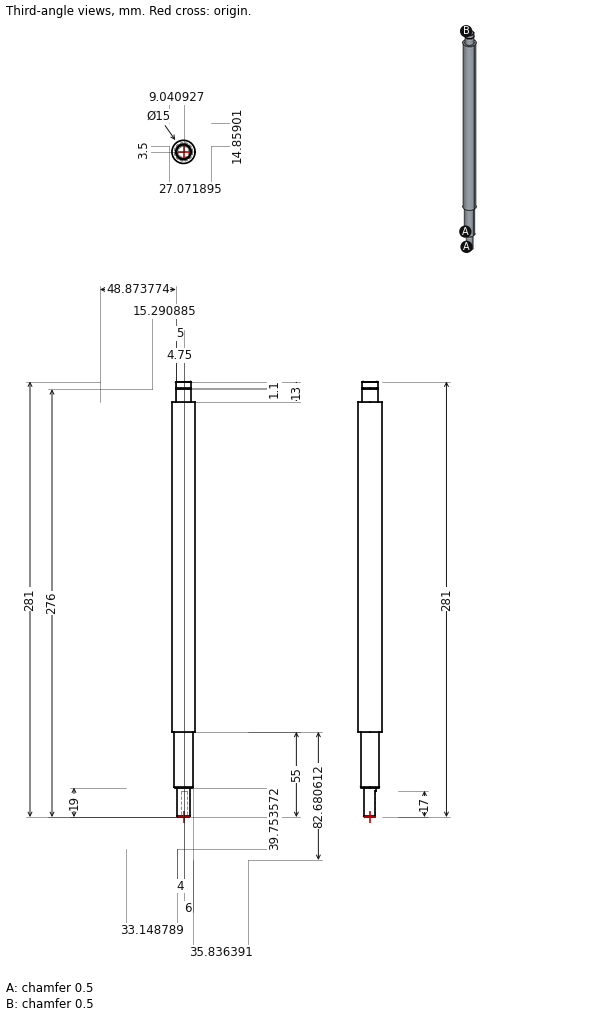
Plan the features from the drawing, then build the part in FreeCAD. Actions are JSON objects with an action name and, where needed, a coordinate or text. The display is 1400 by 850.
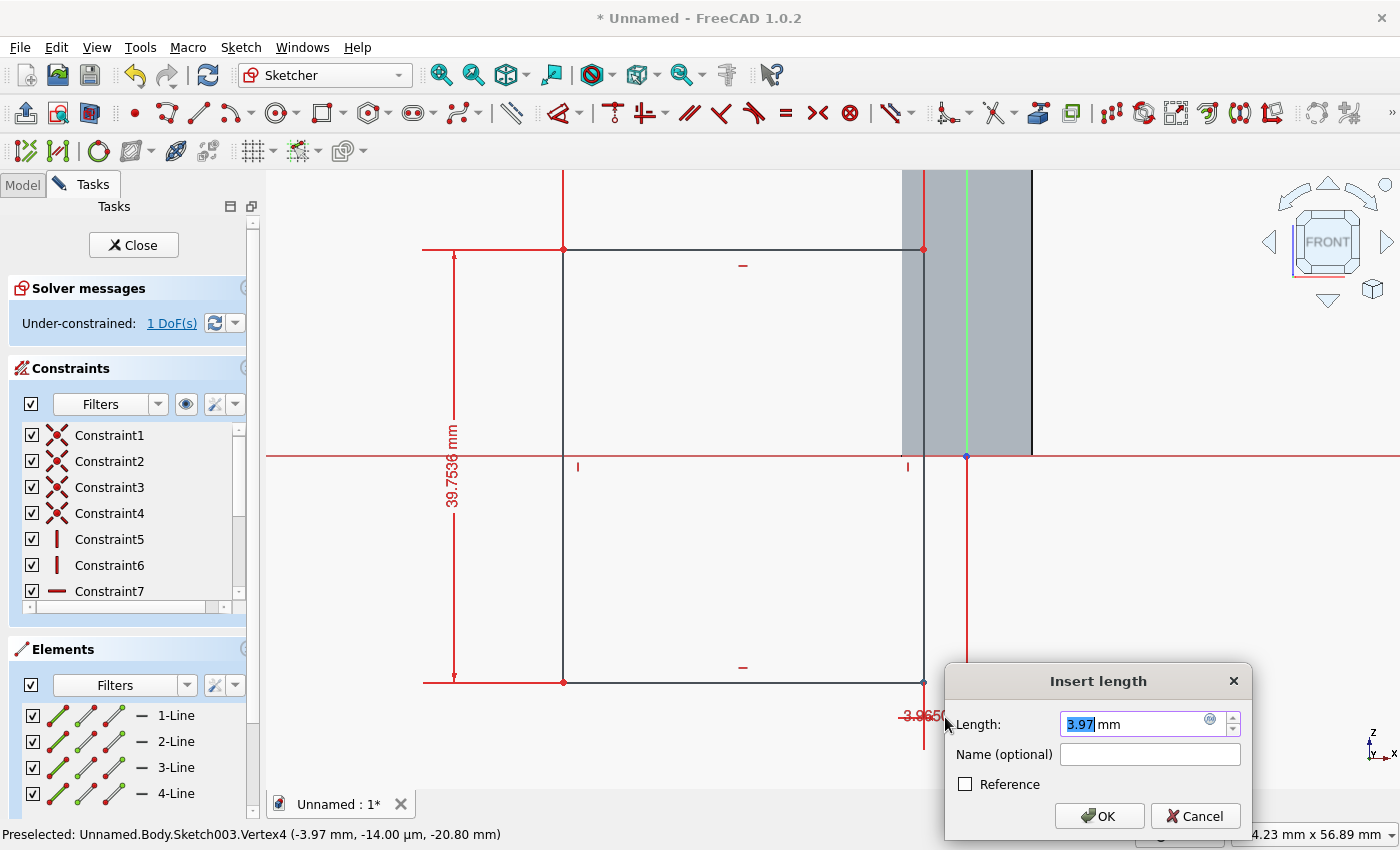
{"action": "type", "text": "4"}
{"action": "key", "text": "Return"}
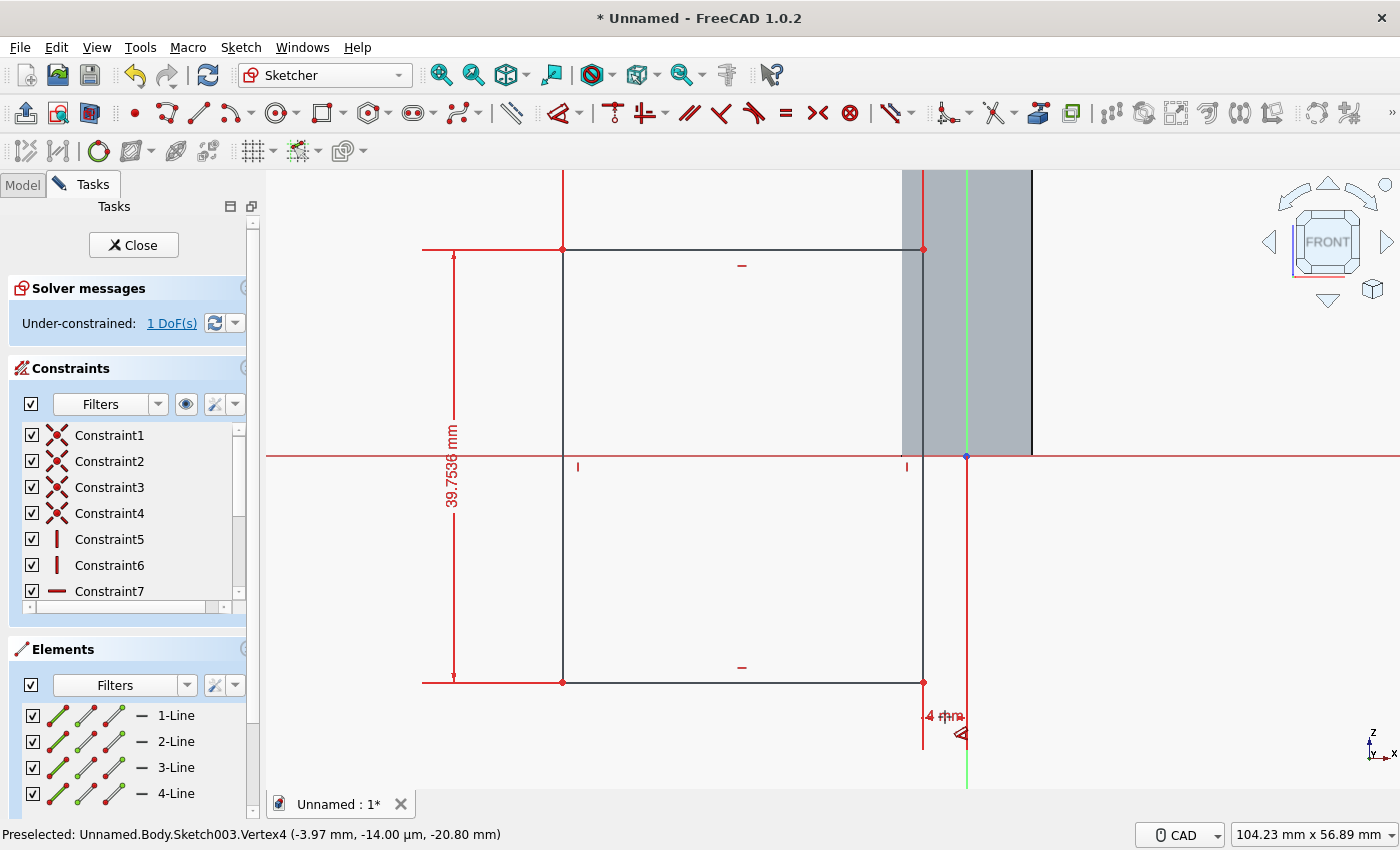
{"action": "left_click", "coordinate": [563, 250]}
{"action": "left_click", "coordinate": [1001, 353]}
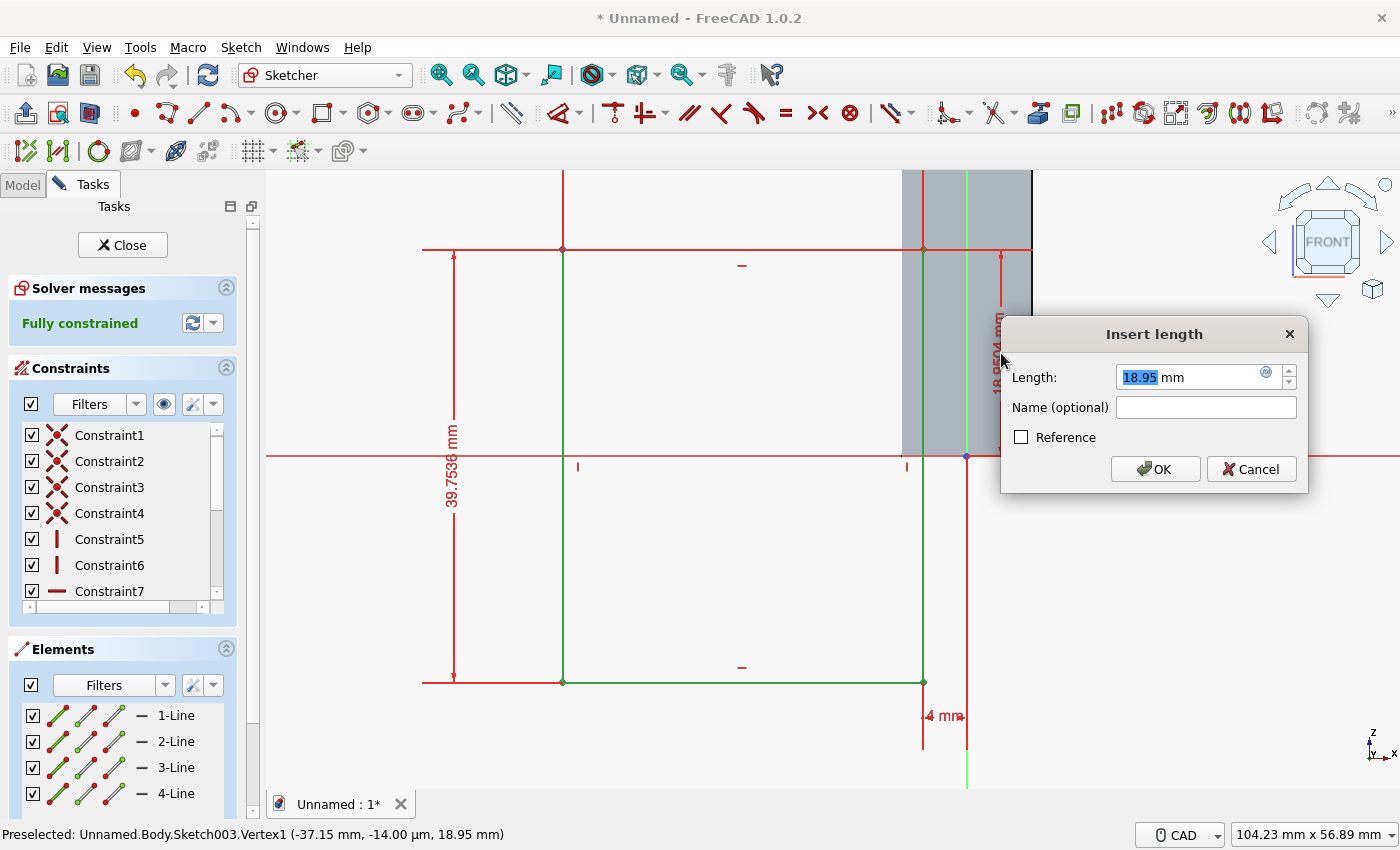
{"action": "type", "text": "19"}
{"action": "key", "text": "Return"}
{"action": "key", "text": "Escape"}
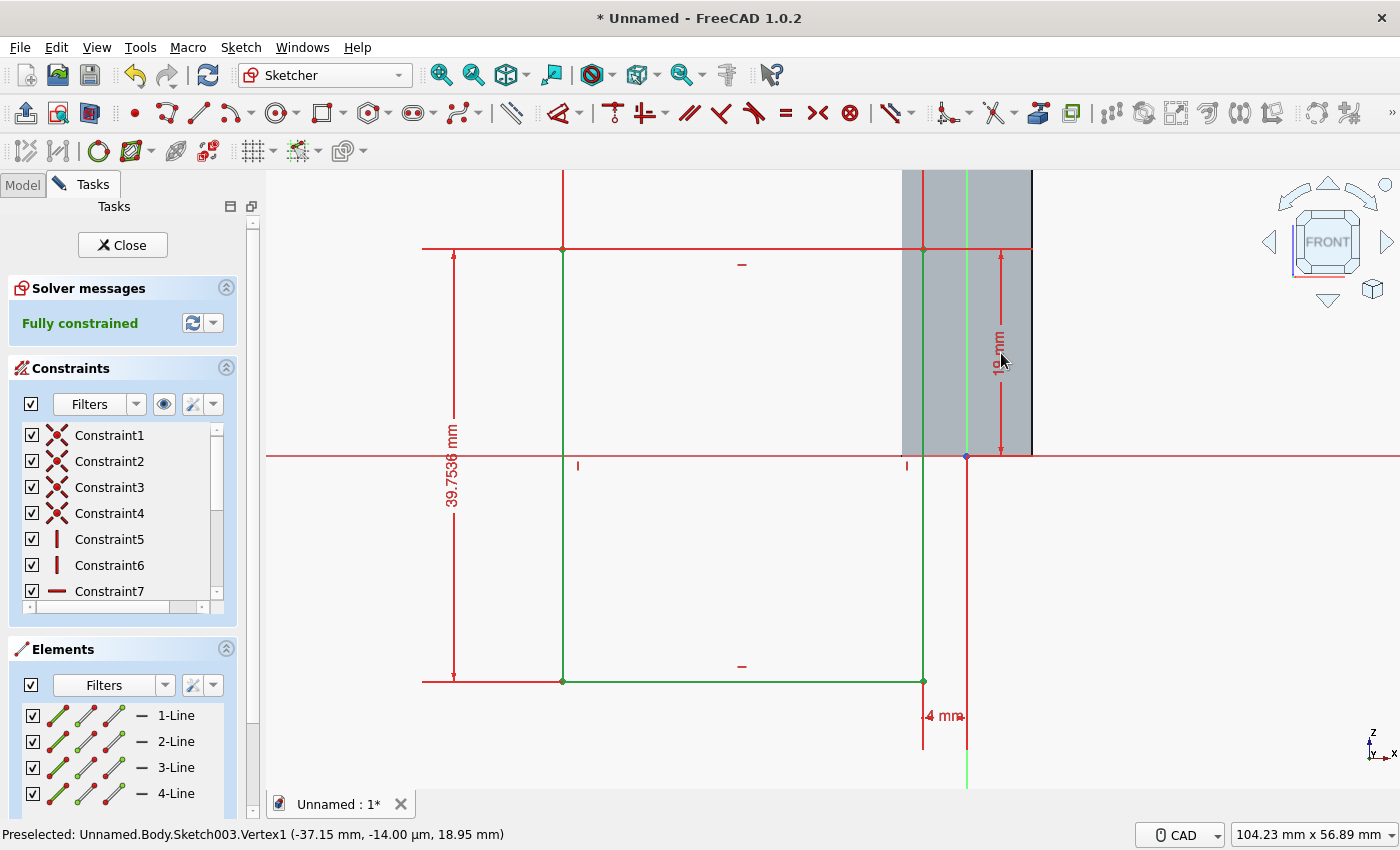
{"action": "left_click", "coordinate": [123, 245]}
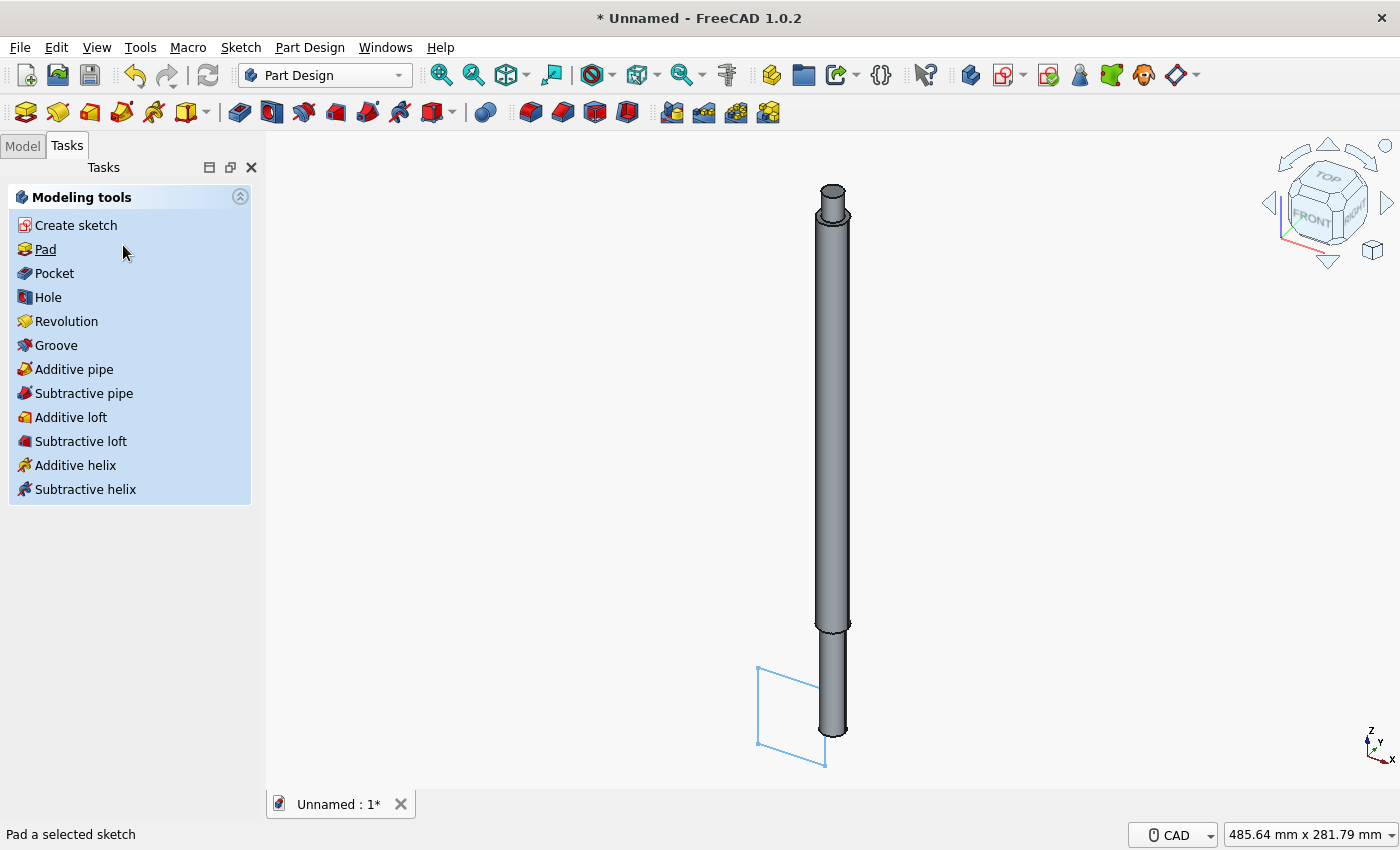
{"action": "left_click", "coordinate": [304, 112]}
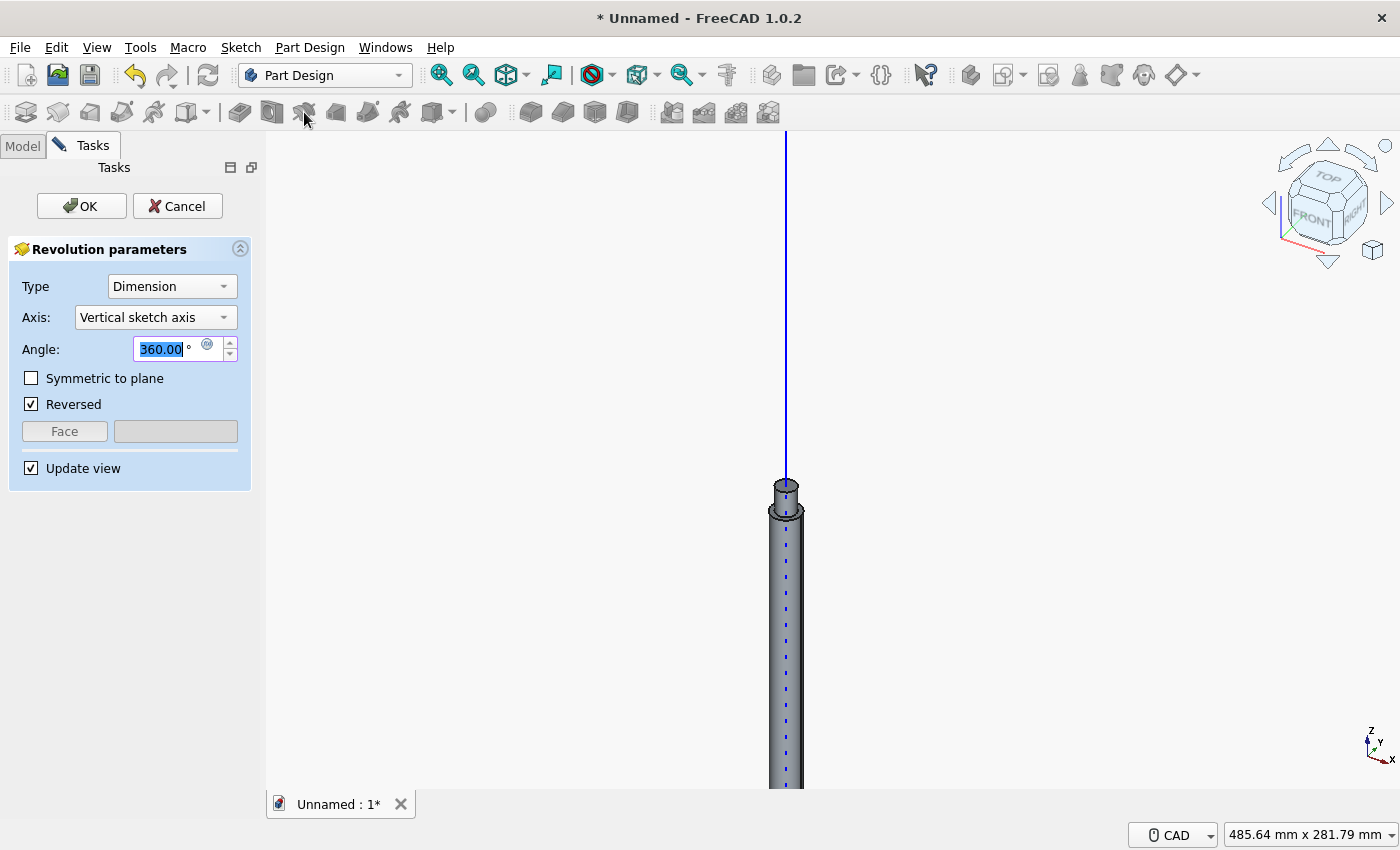
{"action": "left_click", "coordinate": [82, 206]}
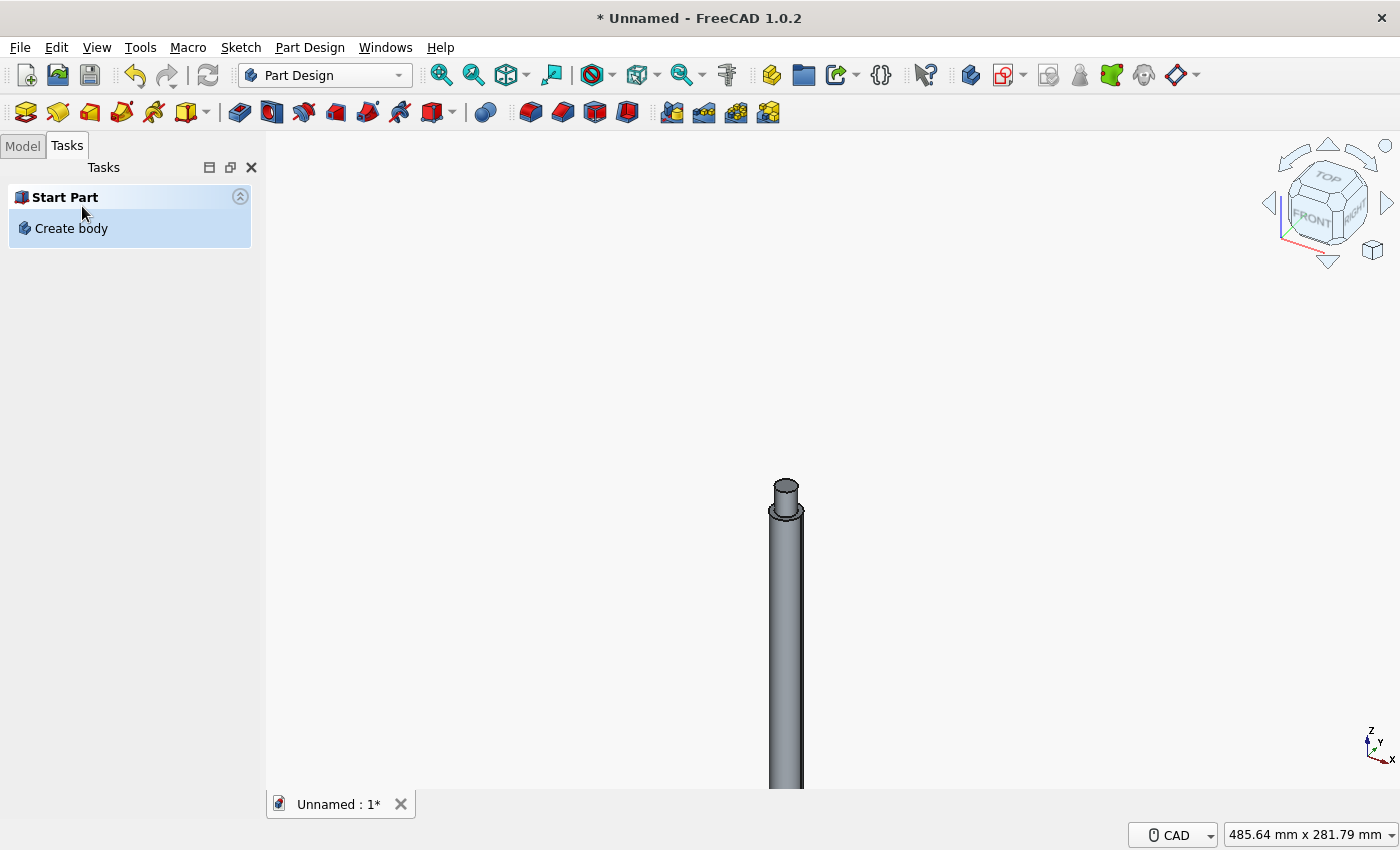
{"action": "left_click", "coordinate": [442, 76]}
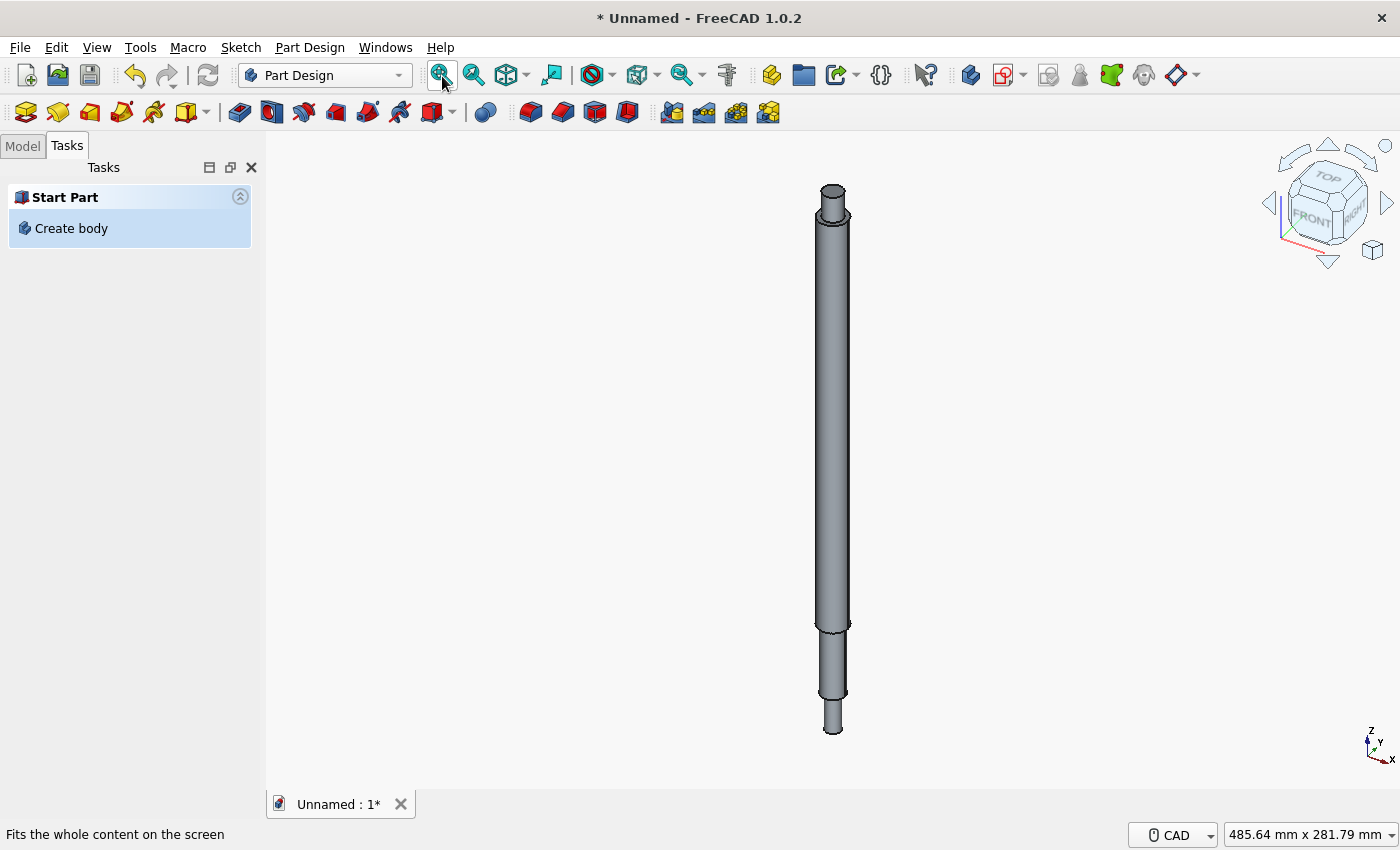
{"action": "left_click", "coordinate": [823, 697]}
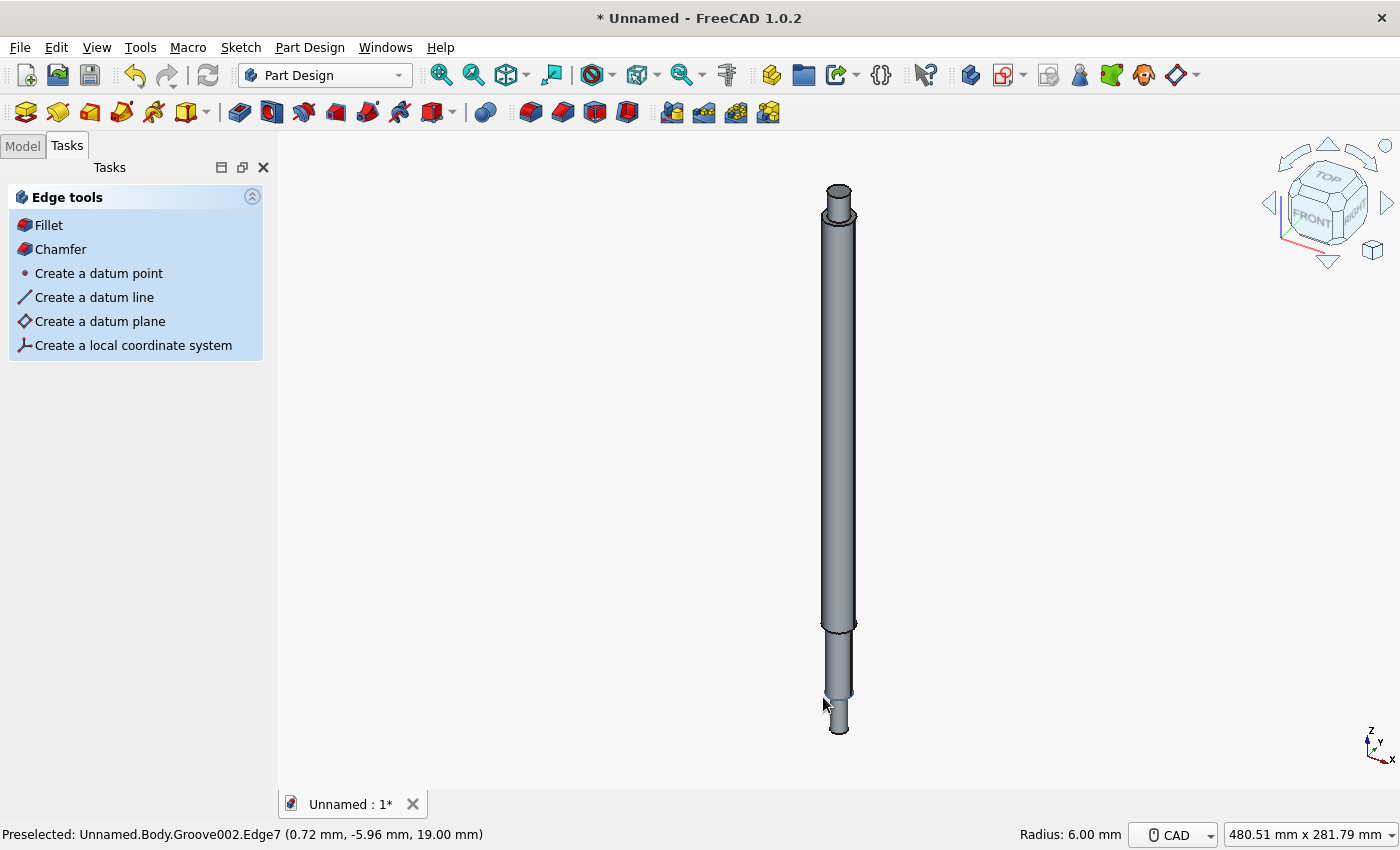
{"action": "left_click", "coordinate": [830, 729], "text": "ctrl"}